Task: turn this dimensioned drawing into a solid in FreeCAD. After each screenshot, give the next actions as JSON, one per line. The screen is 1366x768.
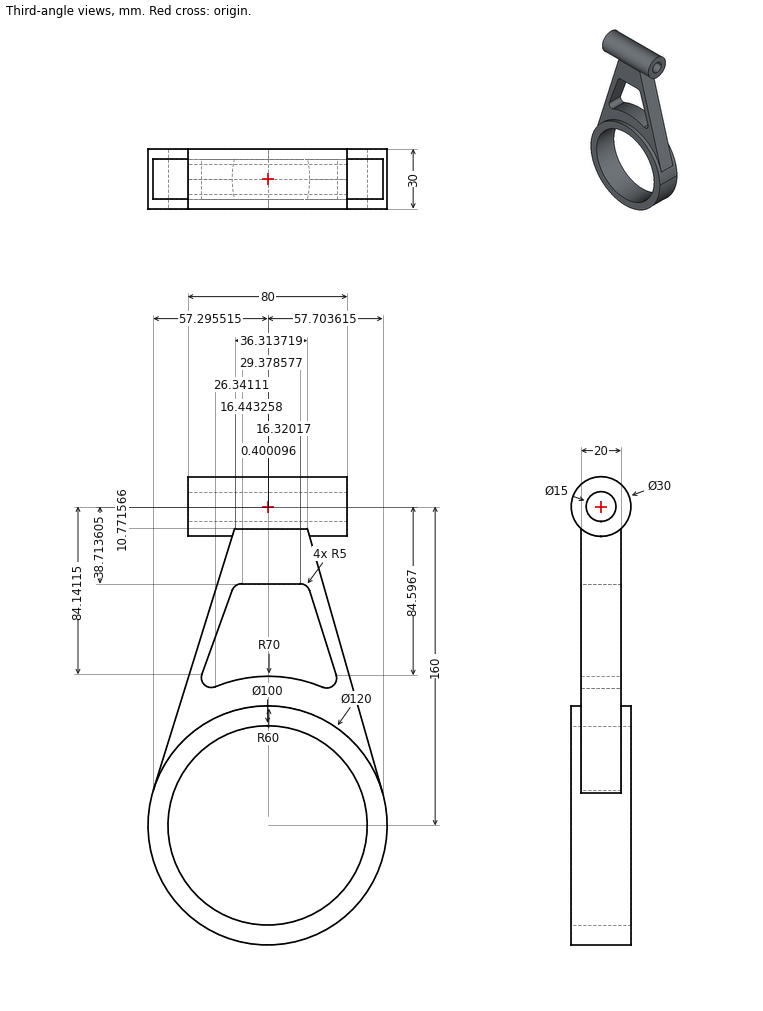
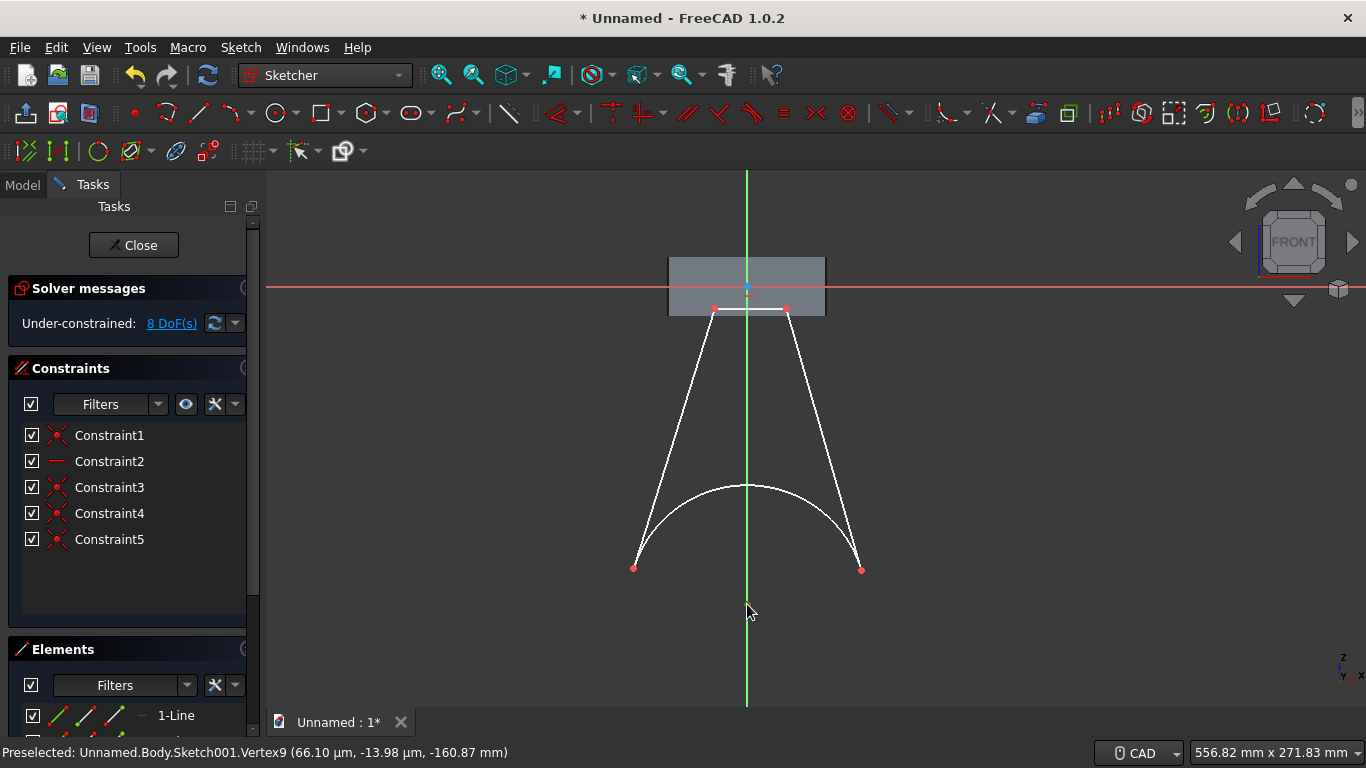
{"action": "left_click", "coordinate": [747, 645]}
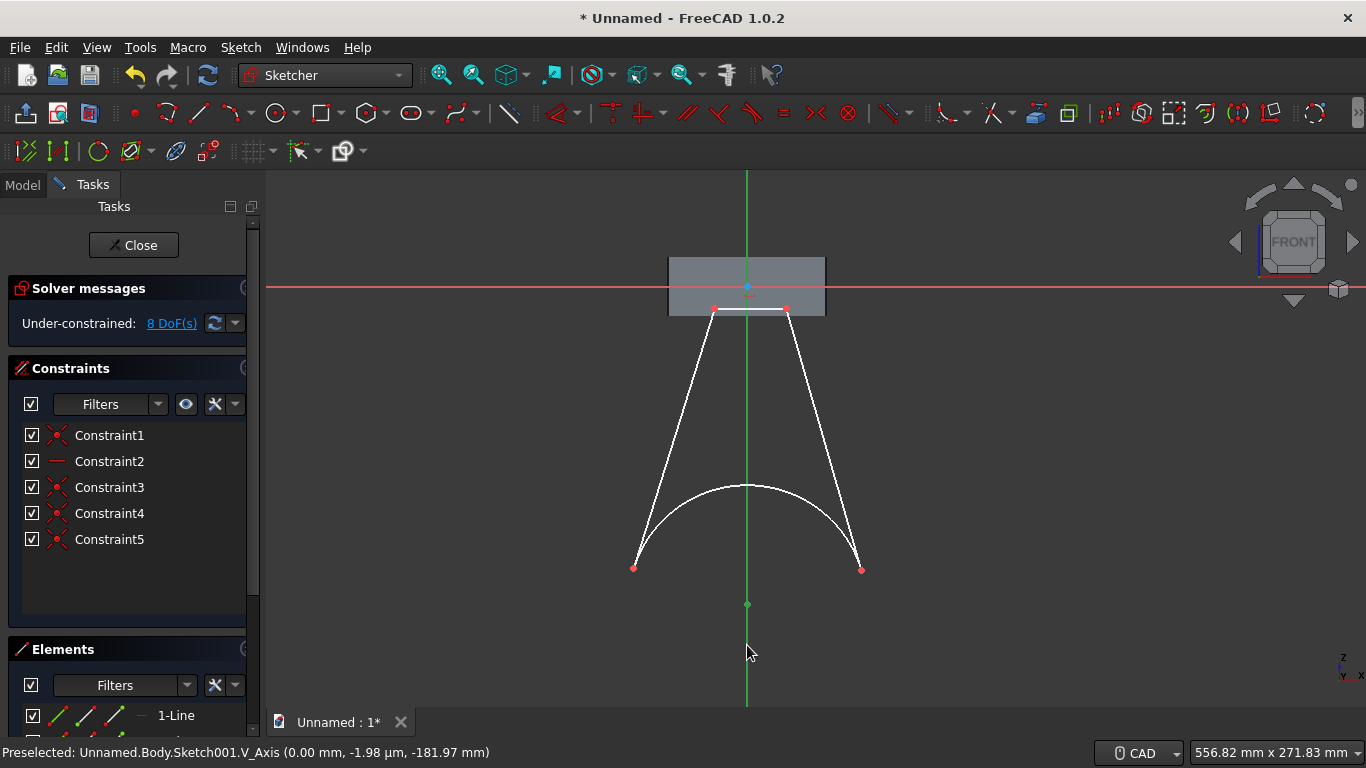
{"action": "left_click", "coordinate": [612, 114]}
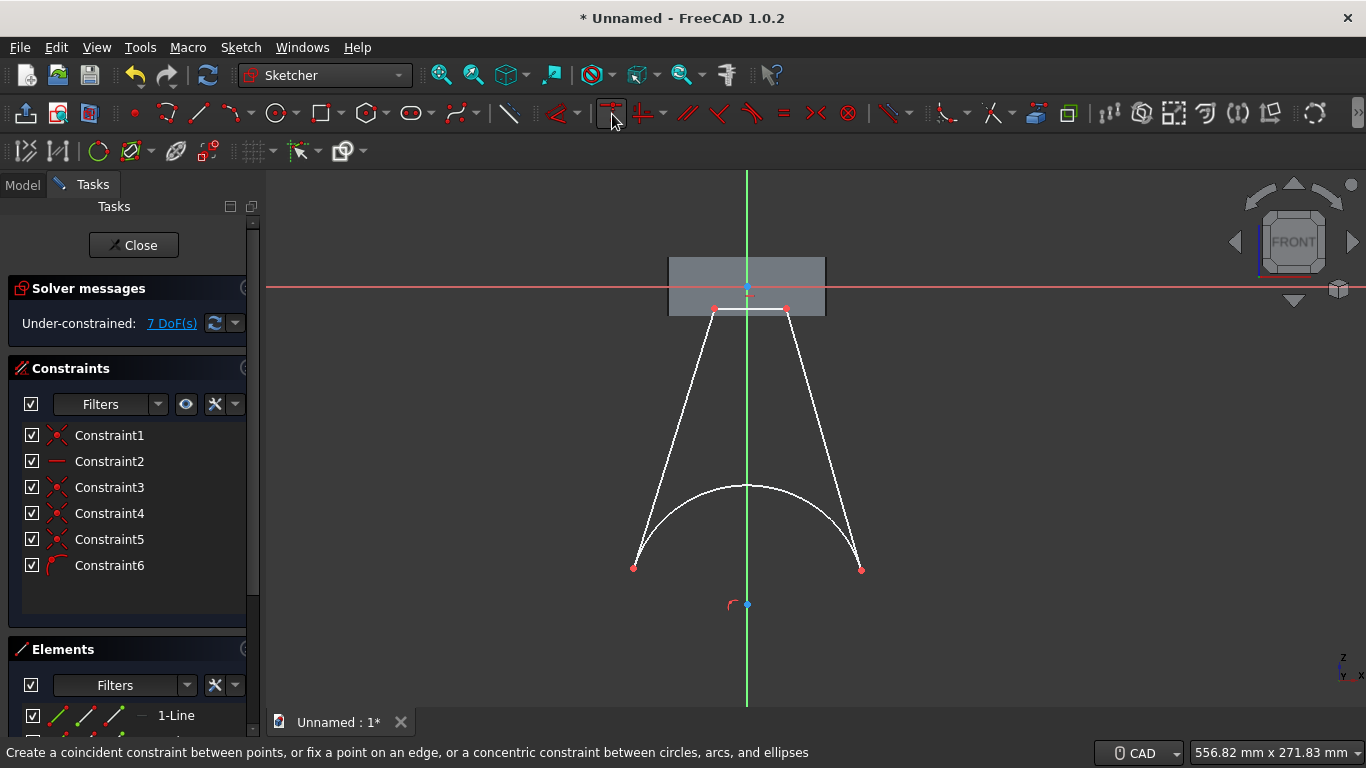
{"action": "left_click", "coordinate": [556, 114]}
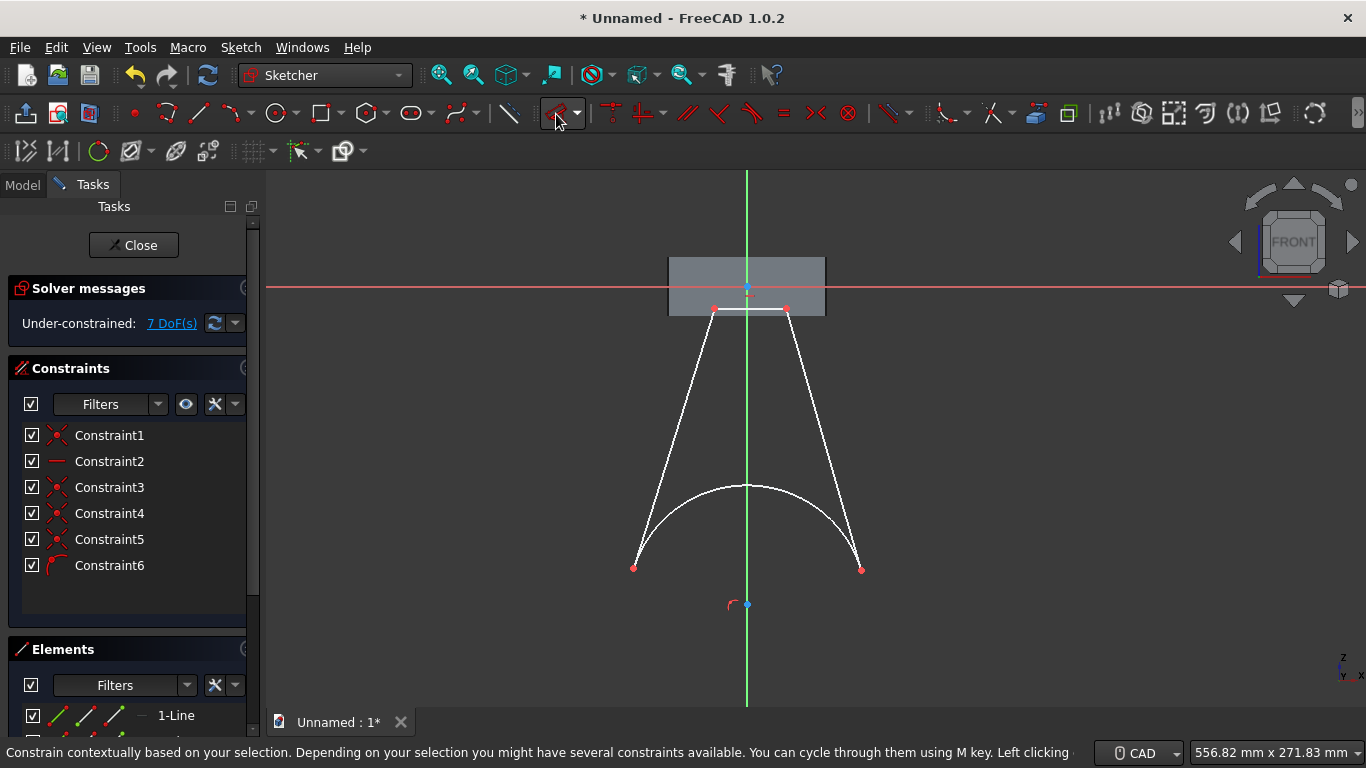
{"action": "left_click", "coordinate": [806, 501]}
{"action": "left_click", "coordinate": [876, 525]}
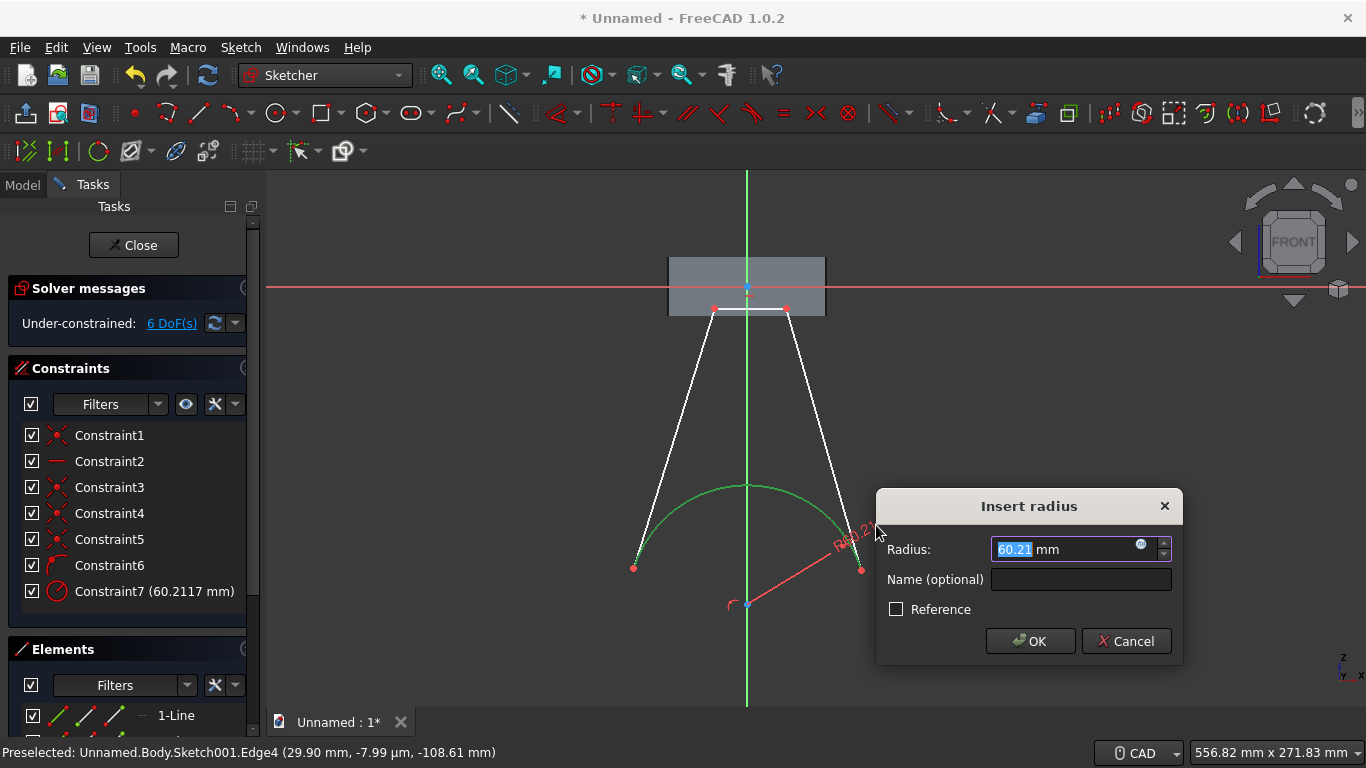
{"action": "type", "text": "60"}
{"action": "key", "text": "Return"}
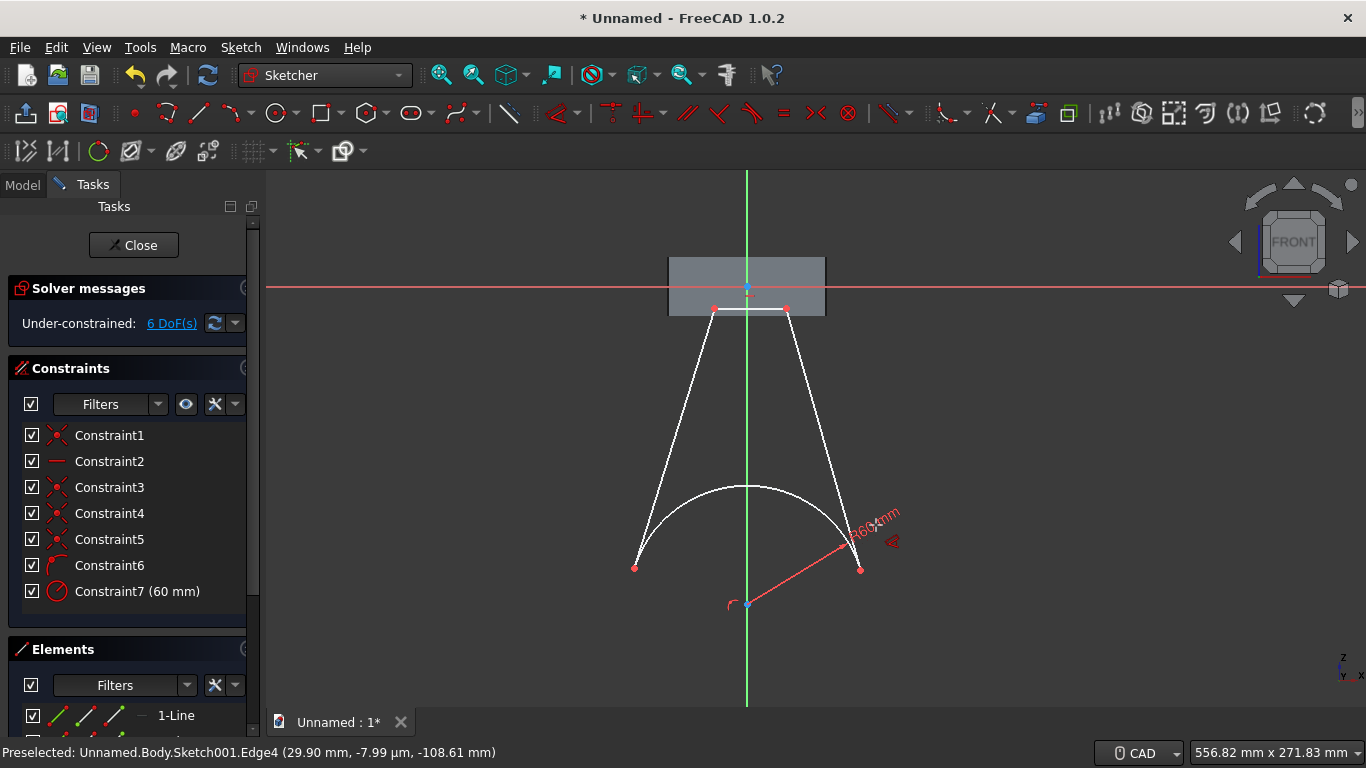
{"action": "left_click", "coordinate": [747, 604]}
{"action": "left_click", "coordinate": [713, 445]}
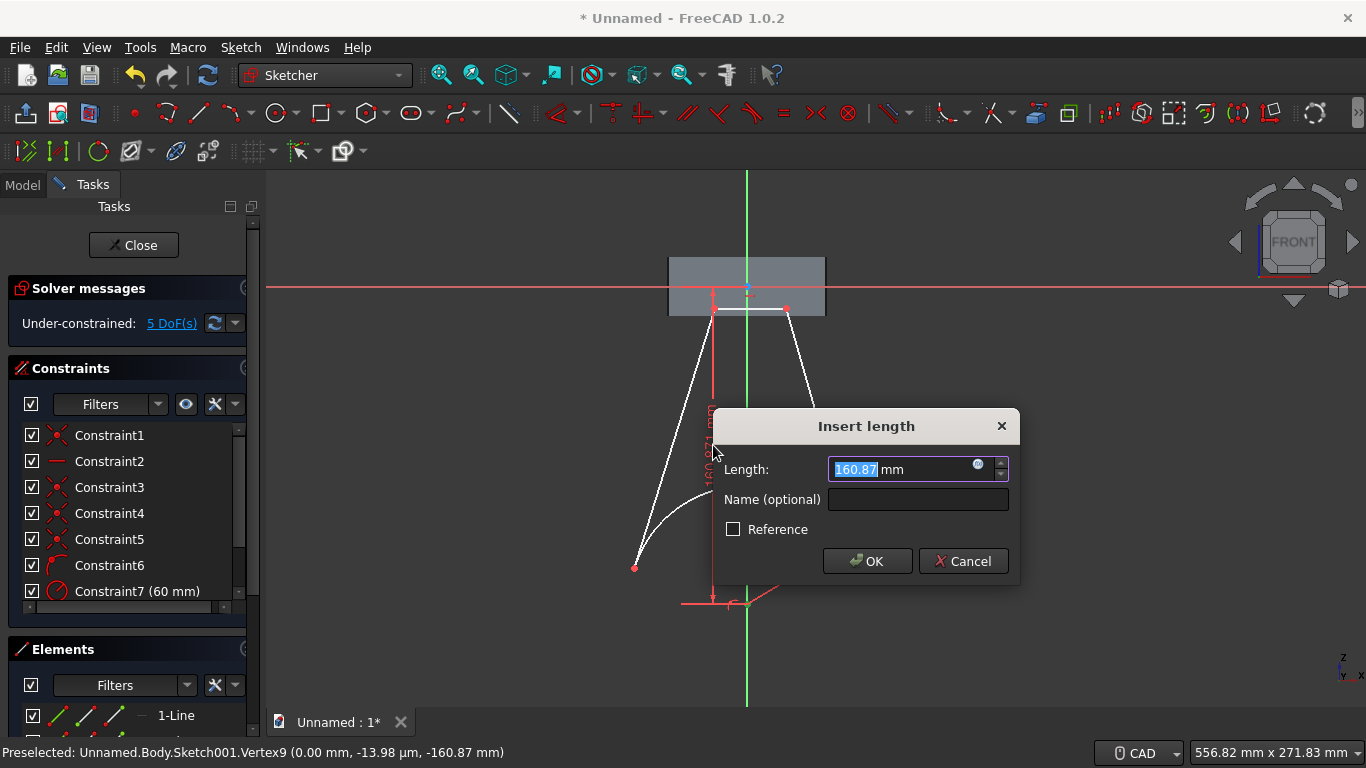
{"action": "type", "text": "160"}
{"action": "key", "text": "Return"}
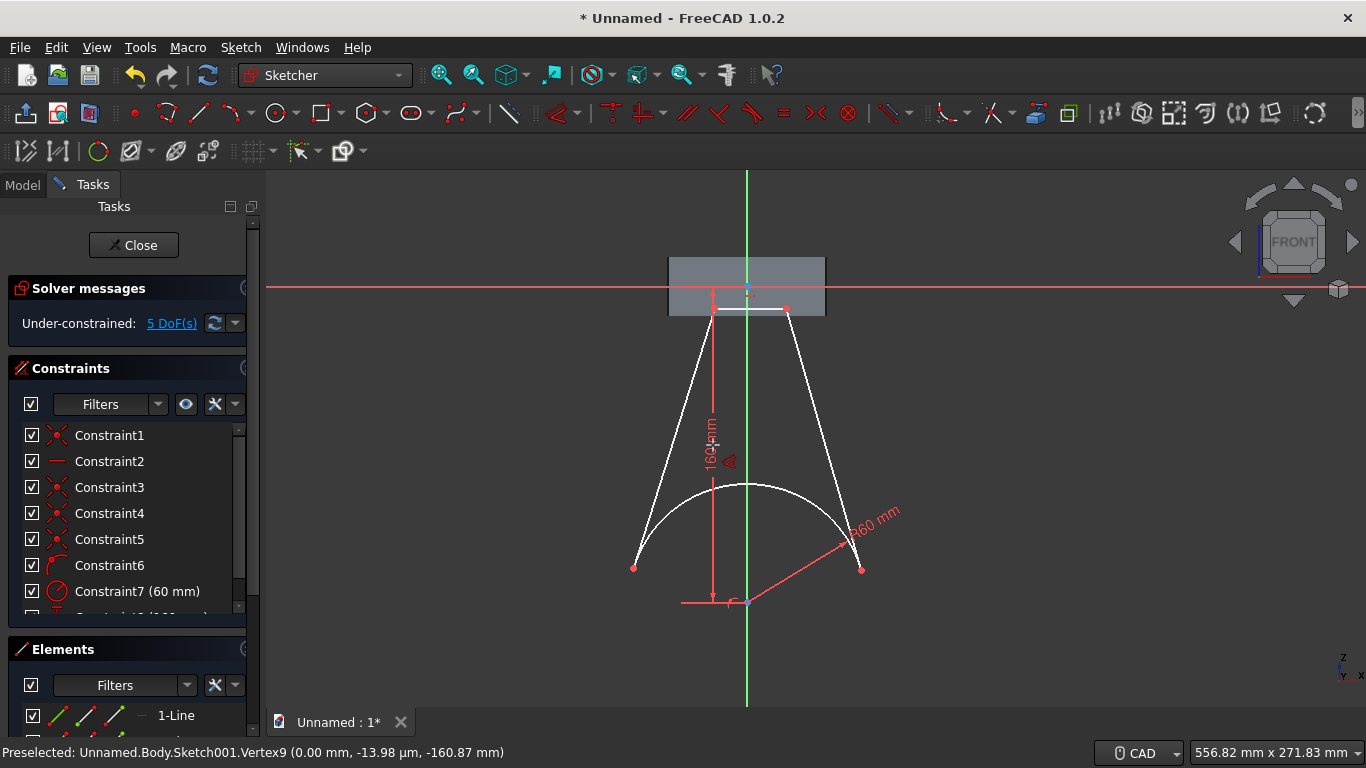
{"action": "scroll", "coordinate": [736, 309], "scroll_direction": "up", "scroll_amount": 2}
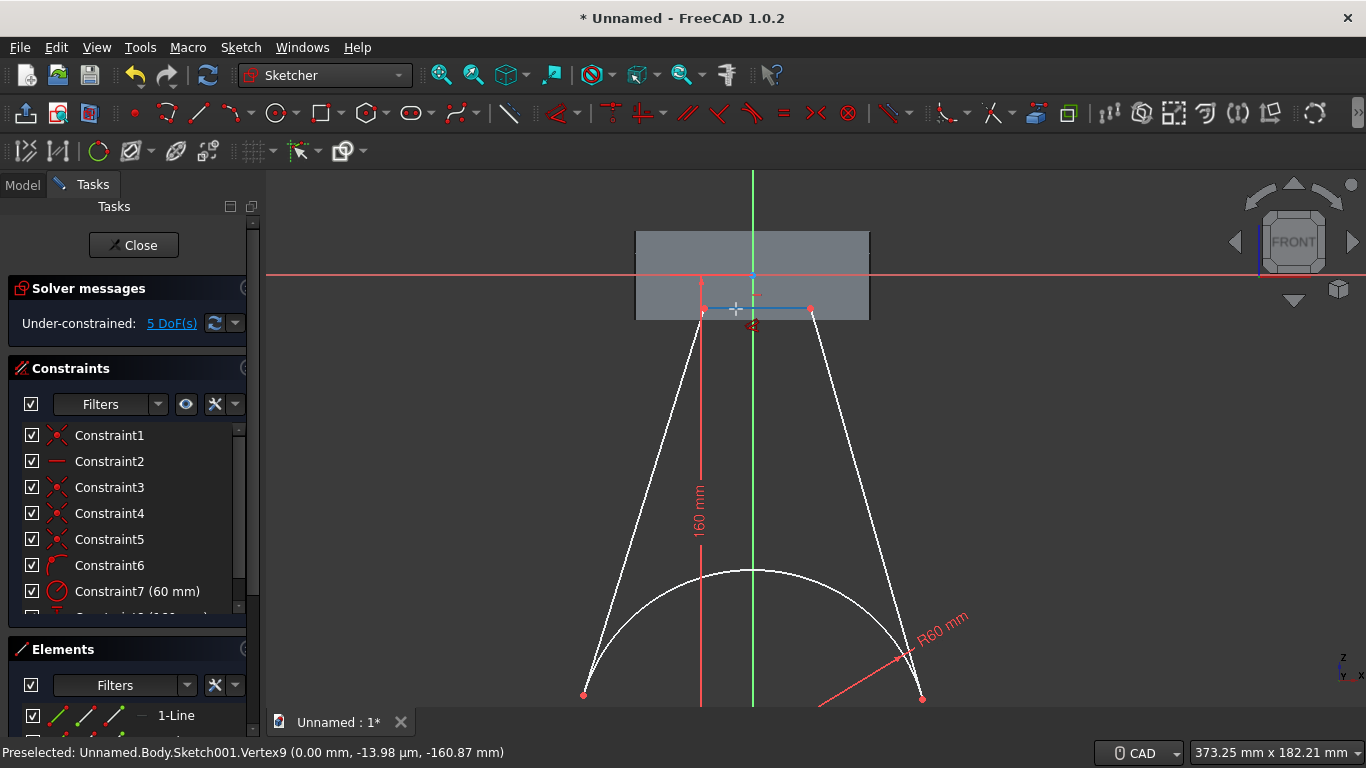
{"action": "left_click", "coordinate": [736, 308]}
{"action": "left_click", "coordinate": [733, 342]}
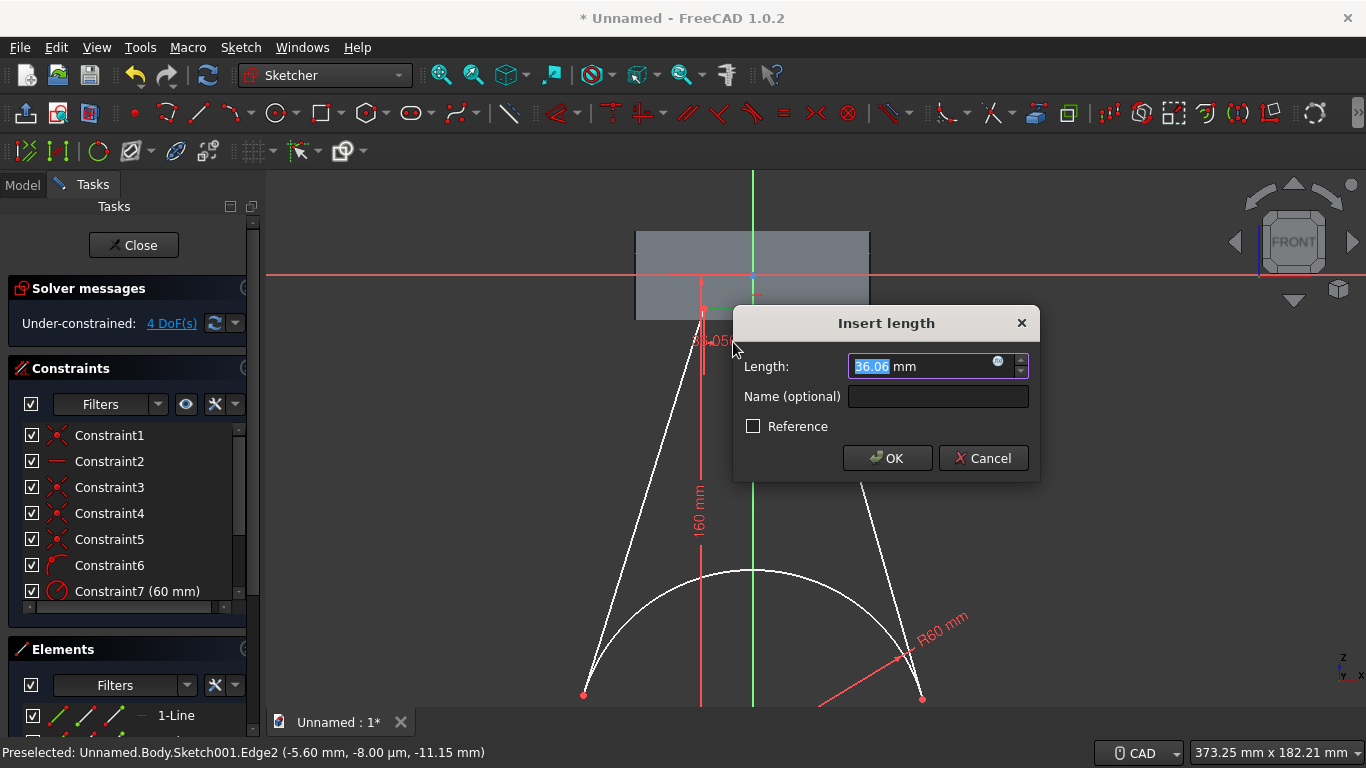
{"action": "type", "text": "36.313719"}
{"action": "key", "text": "Return"}